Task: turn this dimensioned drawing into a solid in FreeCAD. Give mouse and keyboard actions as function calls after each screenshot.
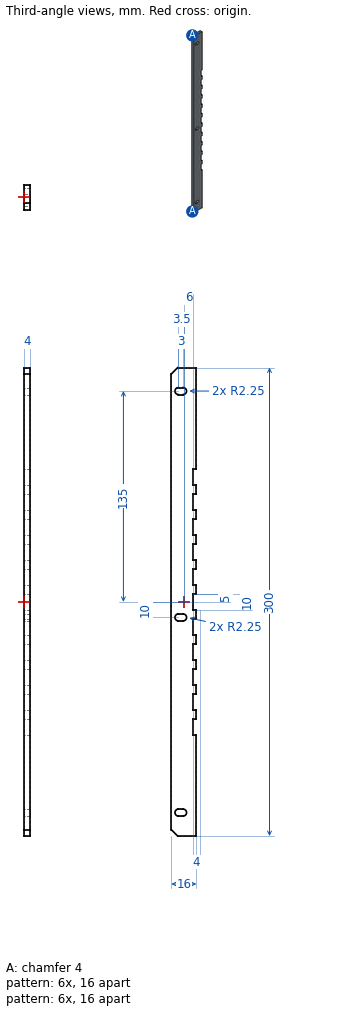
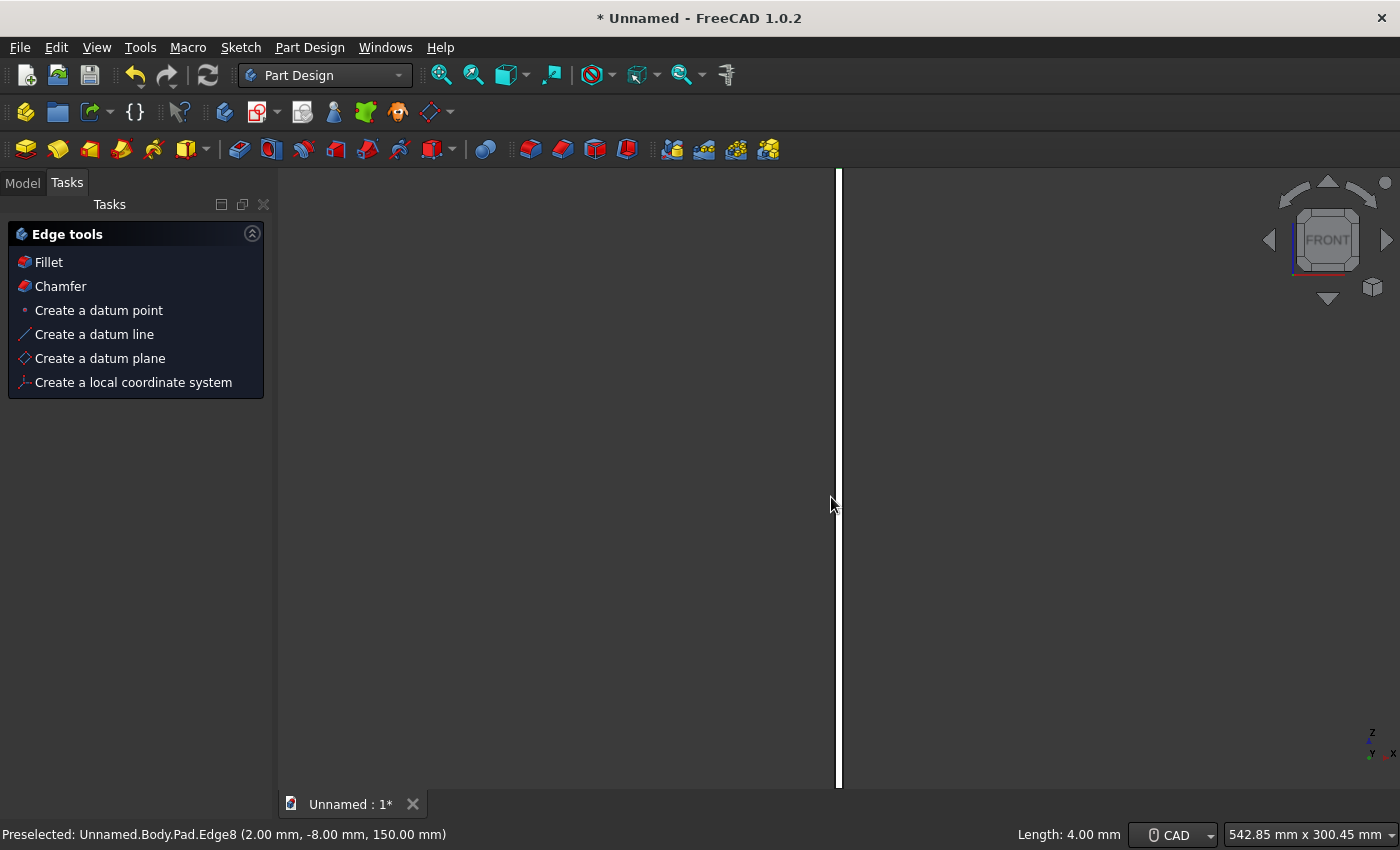
click(442, 76)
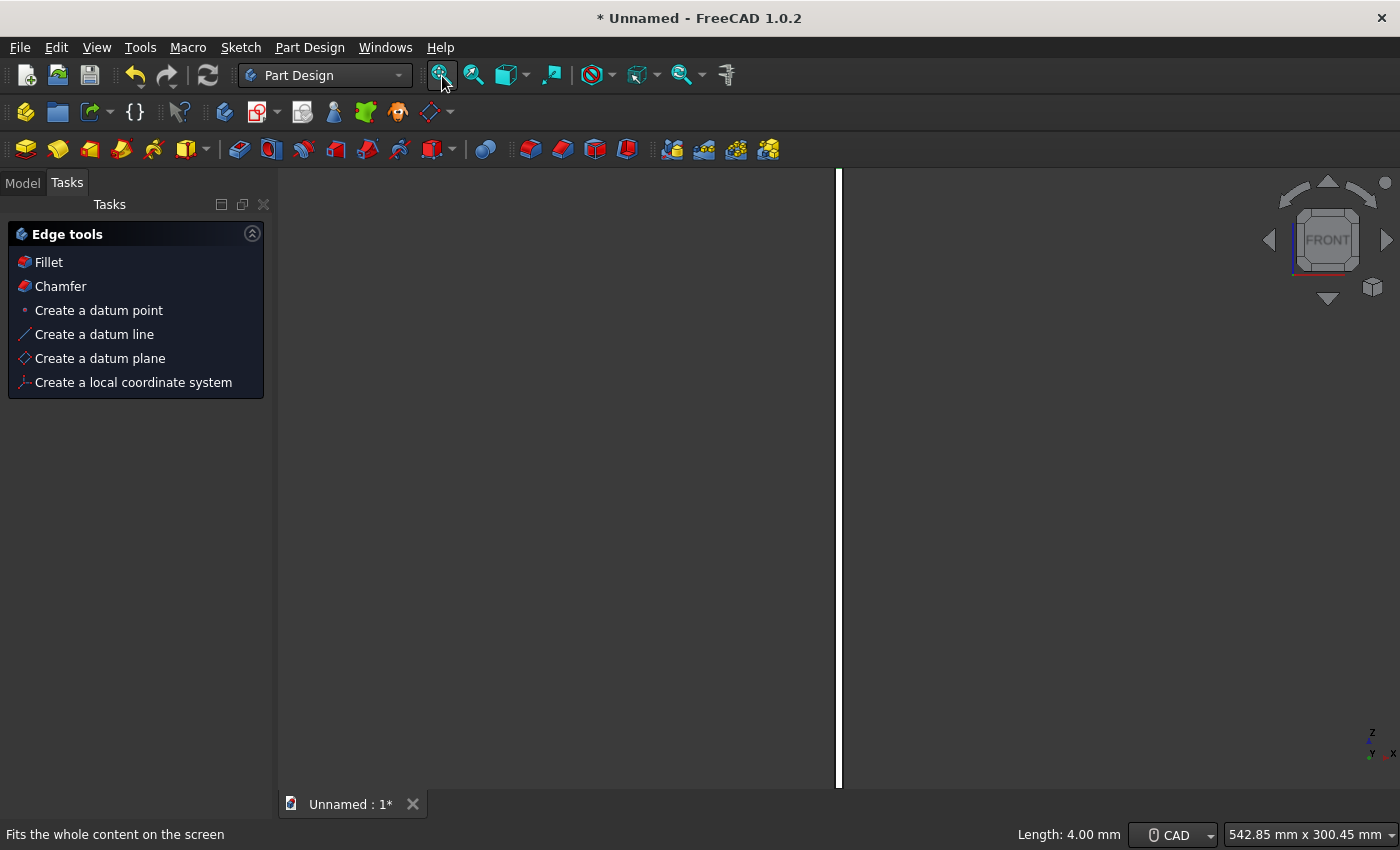
key(3)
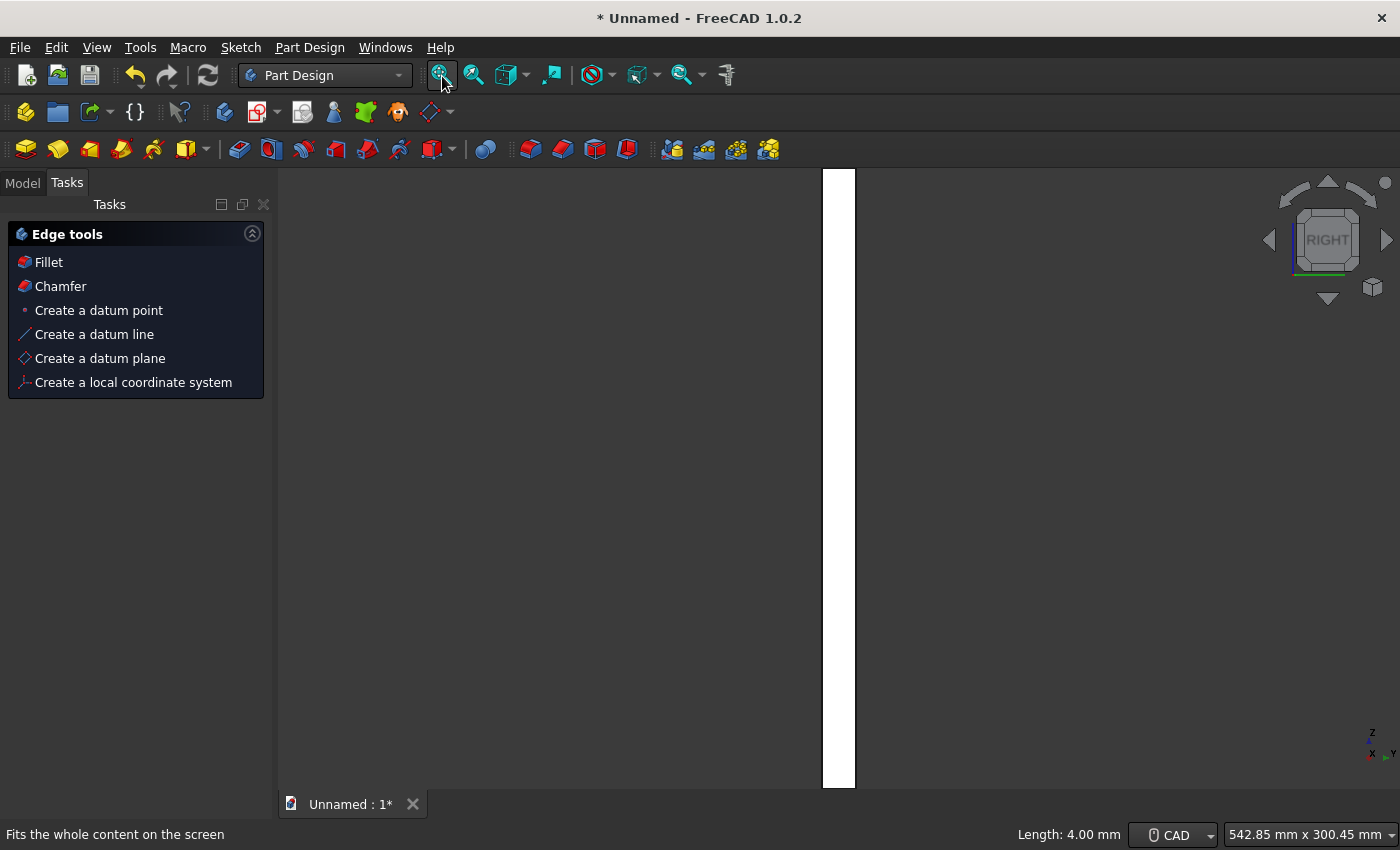
key(v)
key(f)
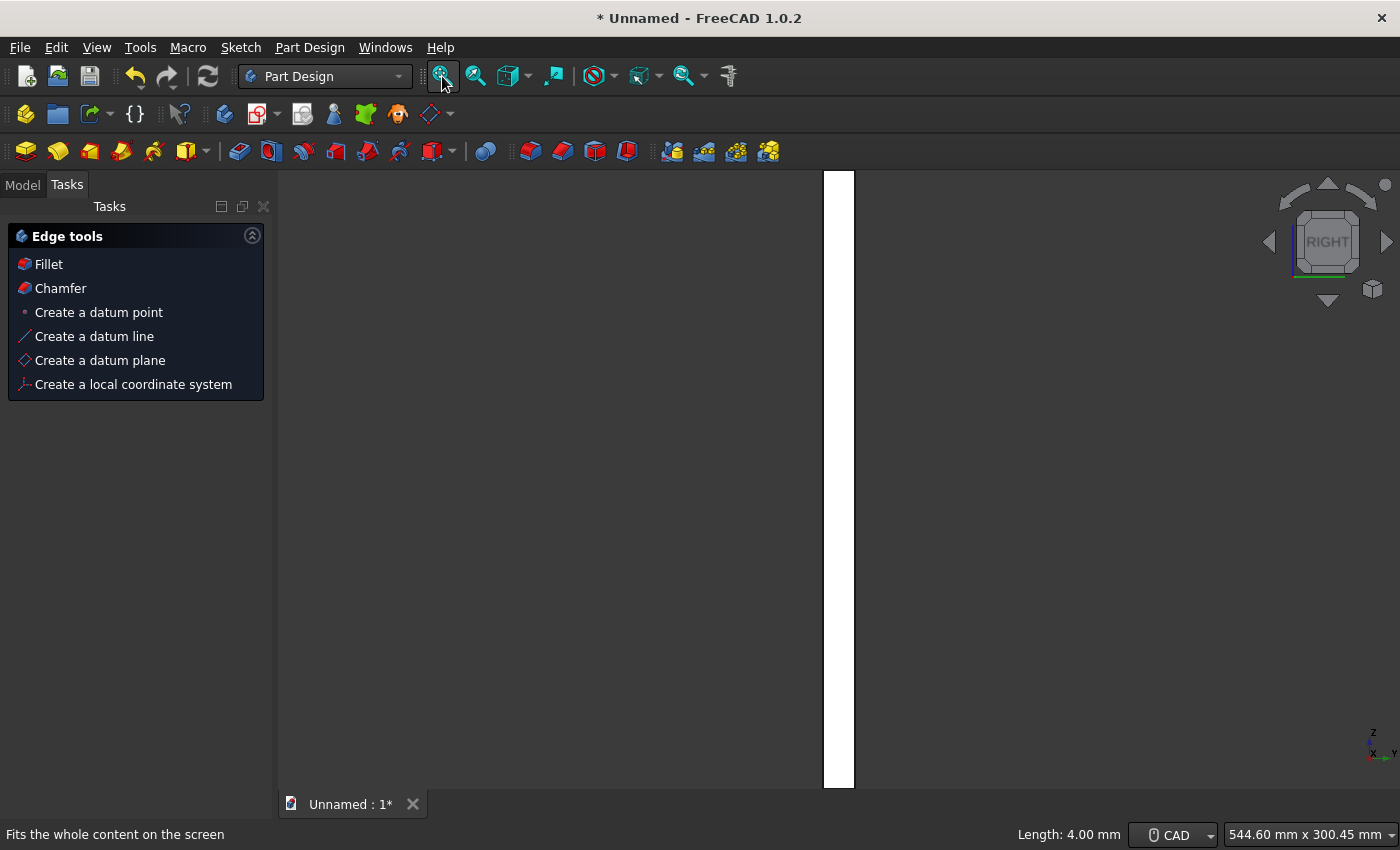
key(5)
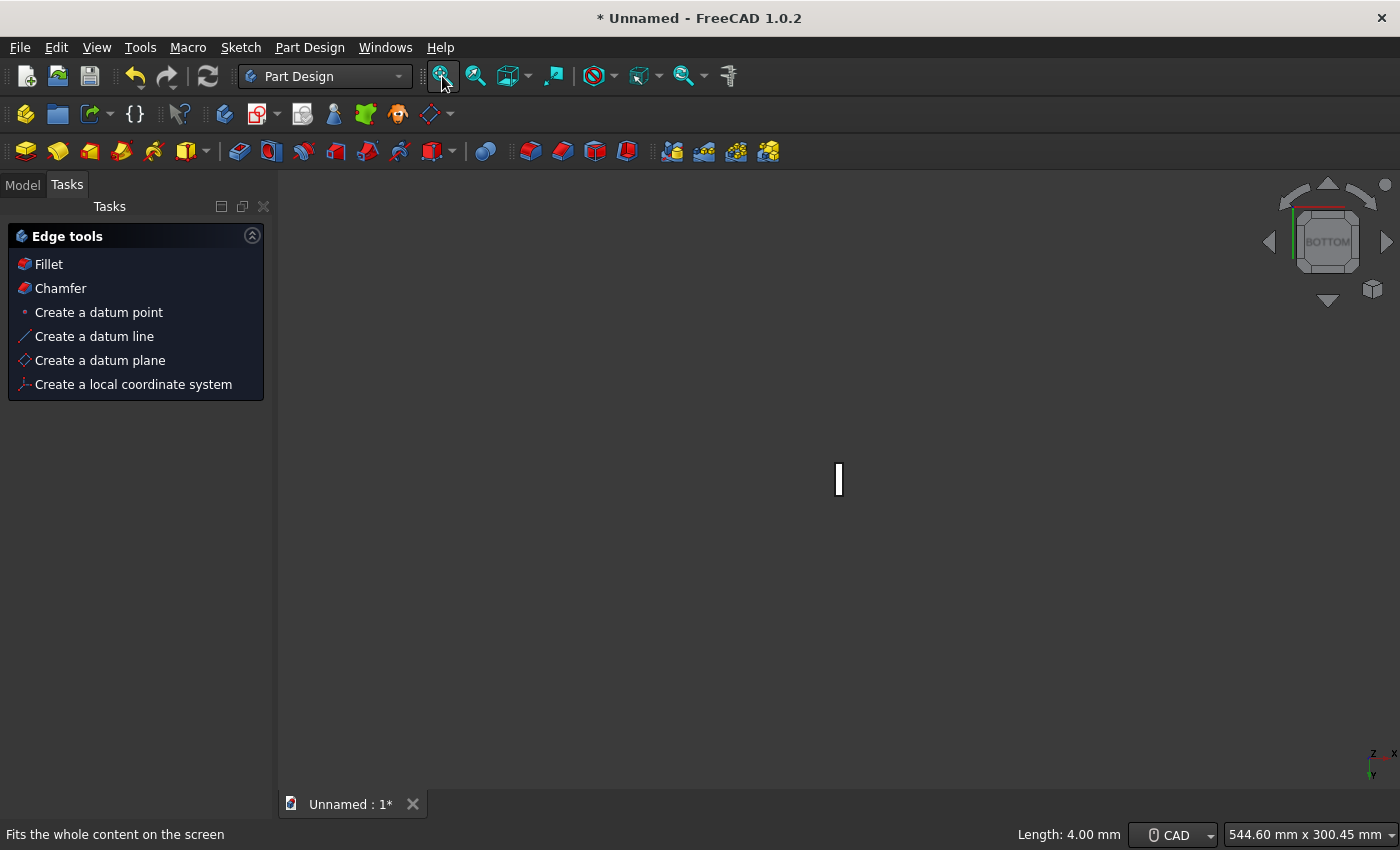
click(444, 76)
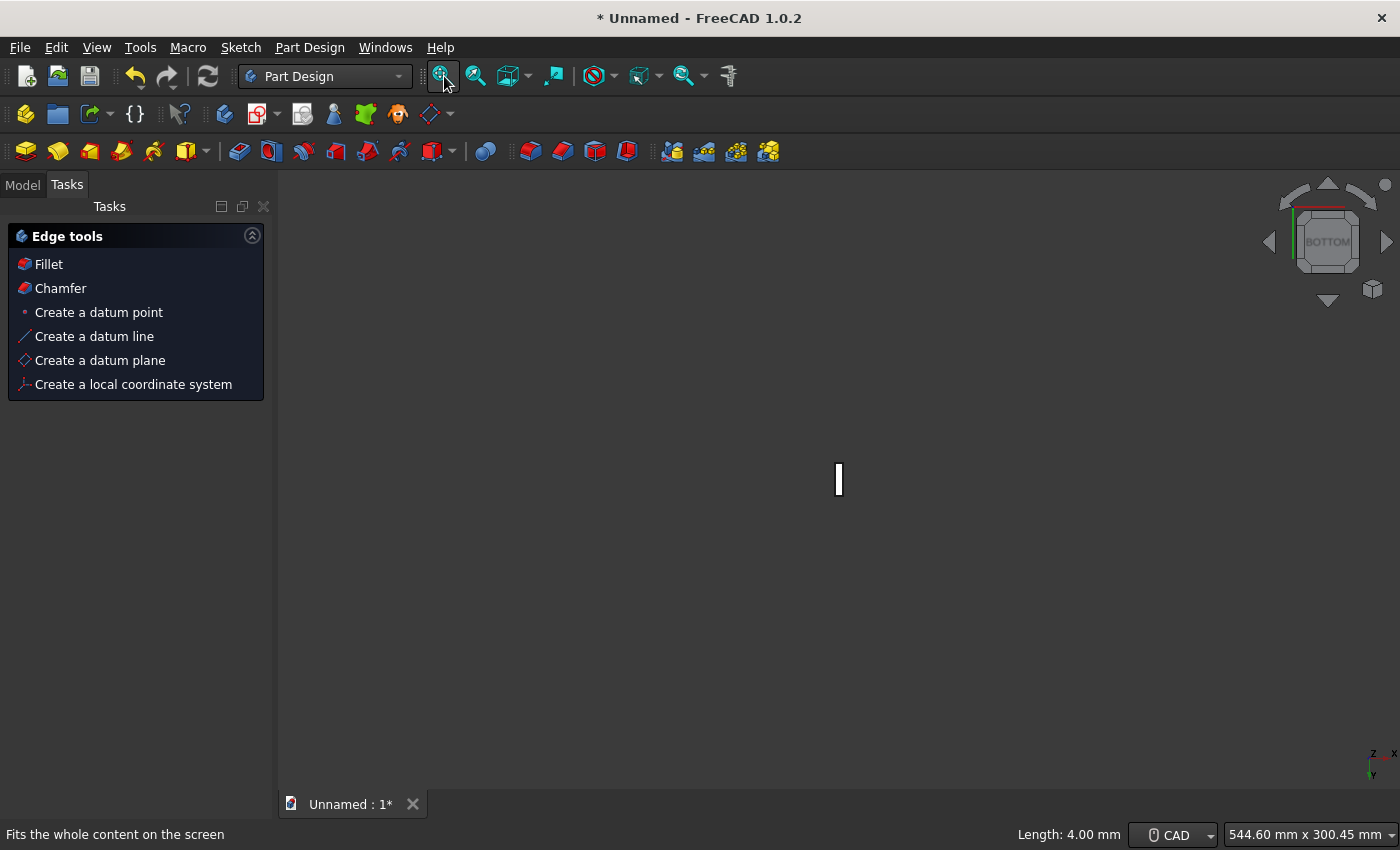
scroll(839, 462, up, 8)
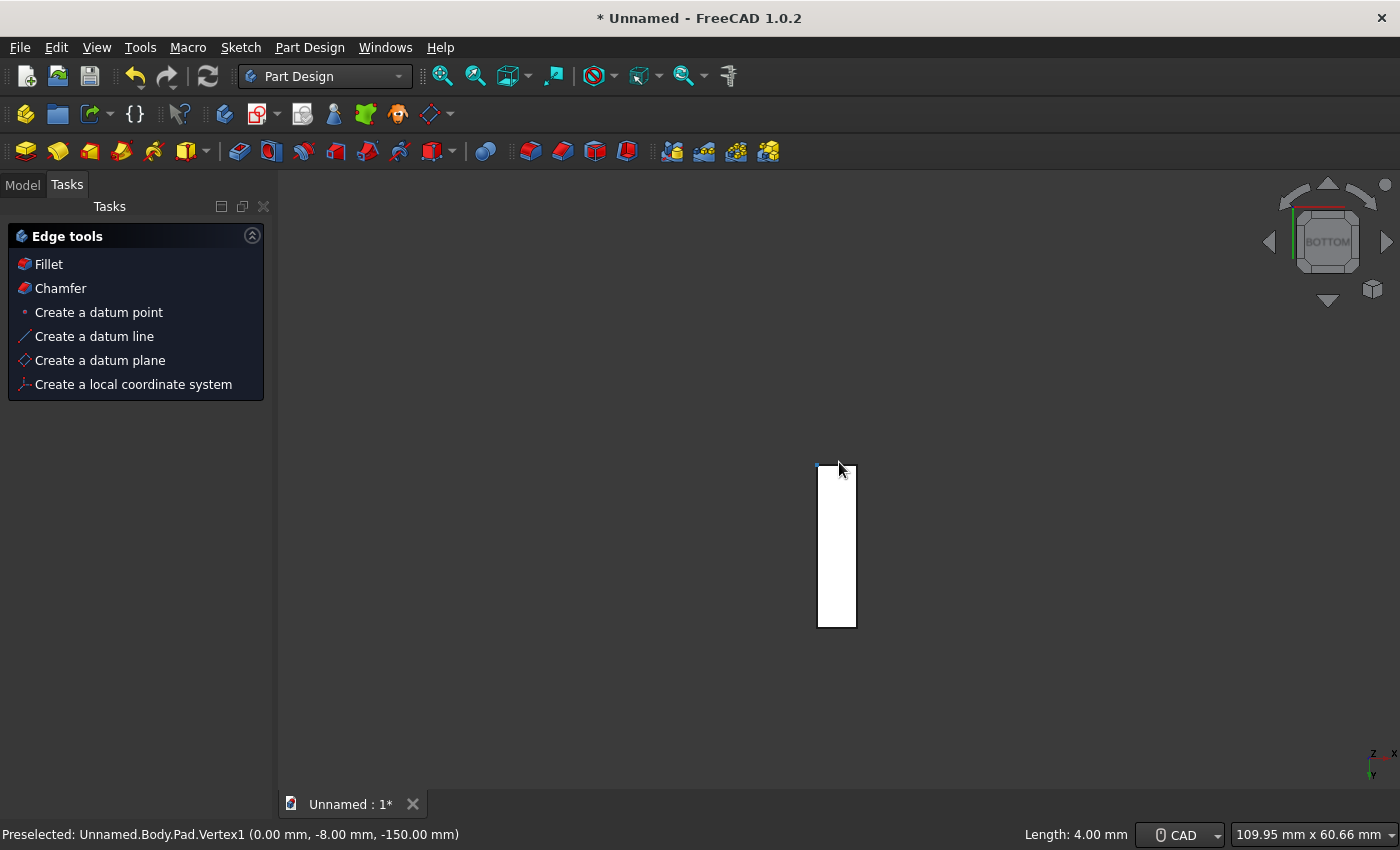
click(837, 464, ctrl)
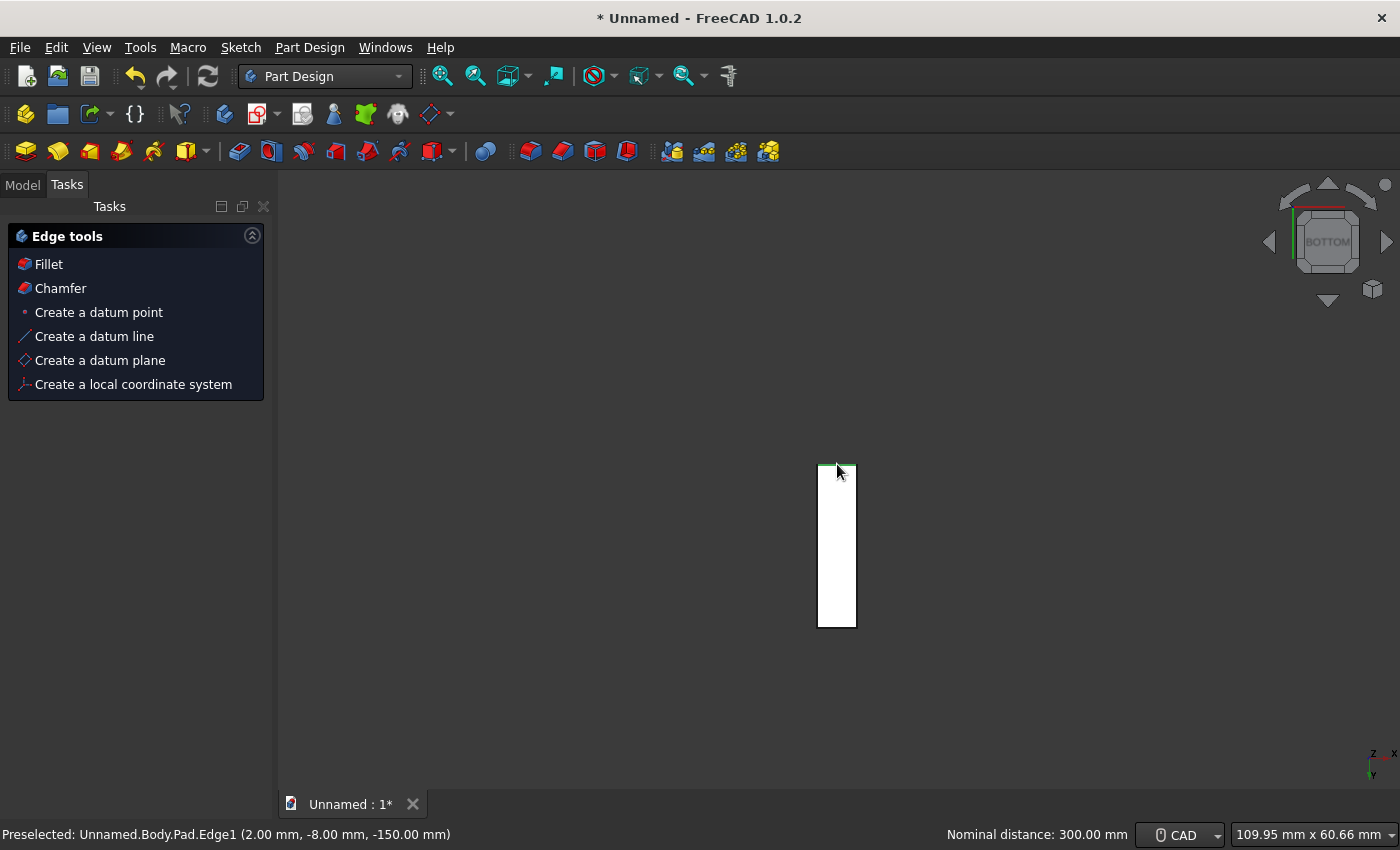
click(564, 152)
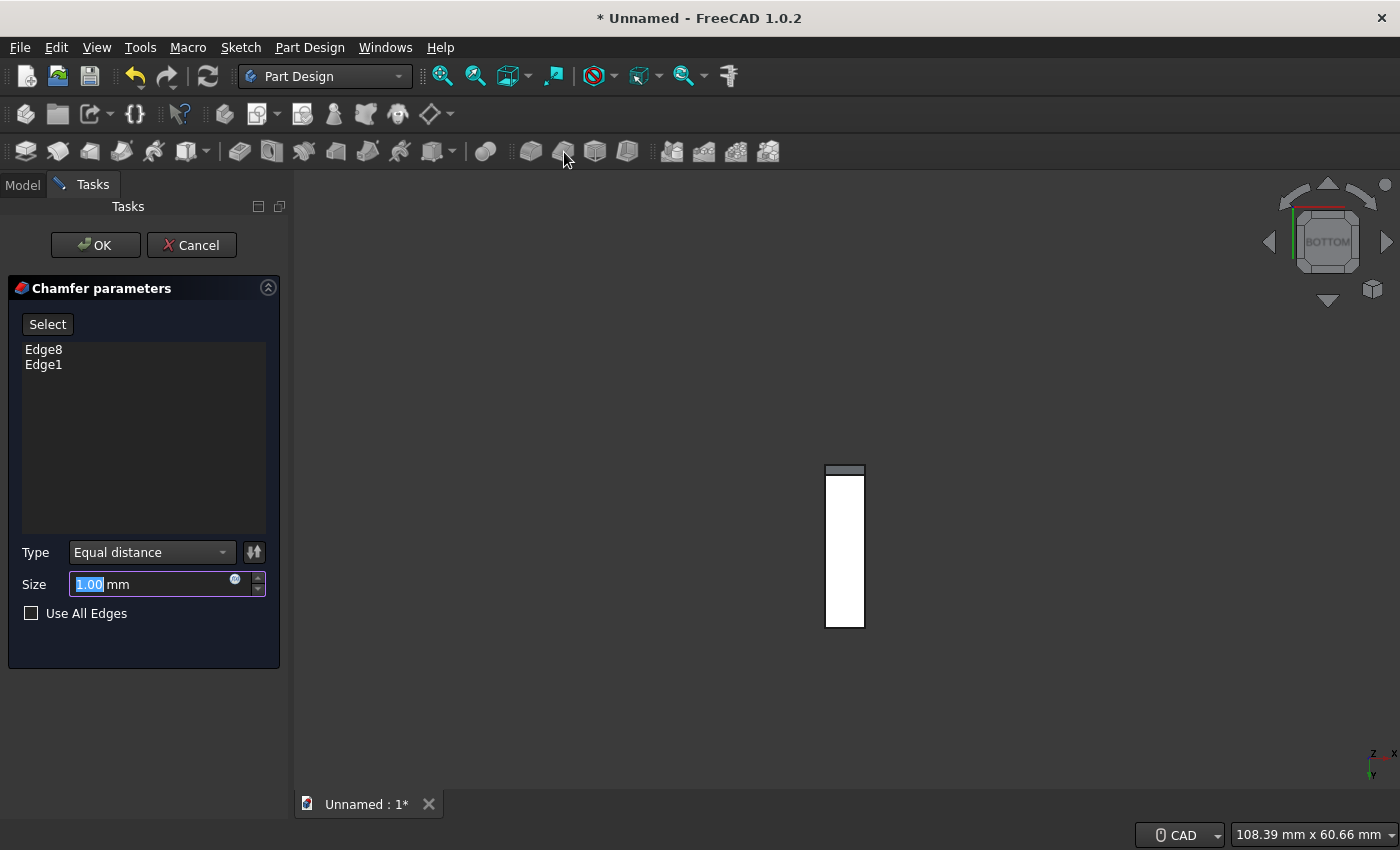
text(4)
key(Tab)